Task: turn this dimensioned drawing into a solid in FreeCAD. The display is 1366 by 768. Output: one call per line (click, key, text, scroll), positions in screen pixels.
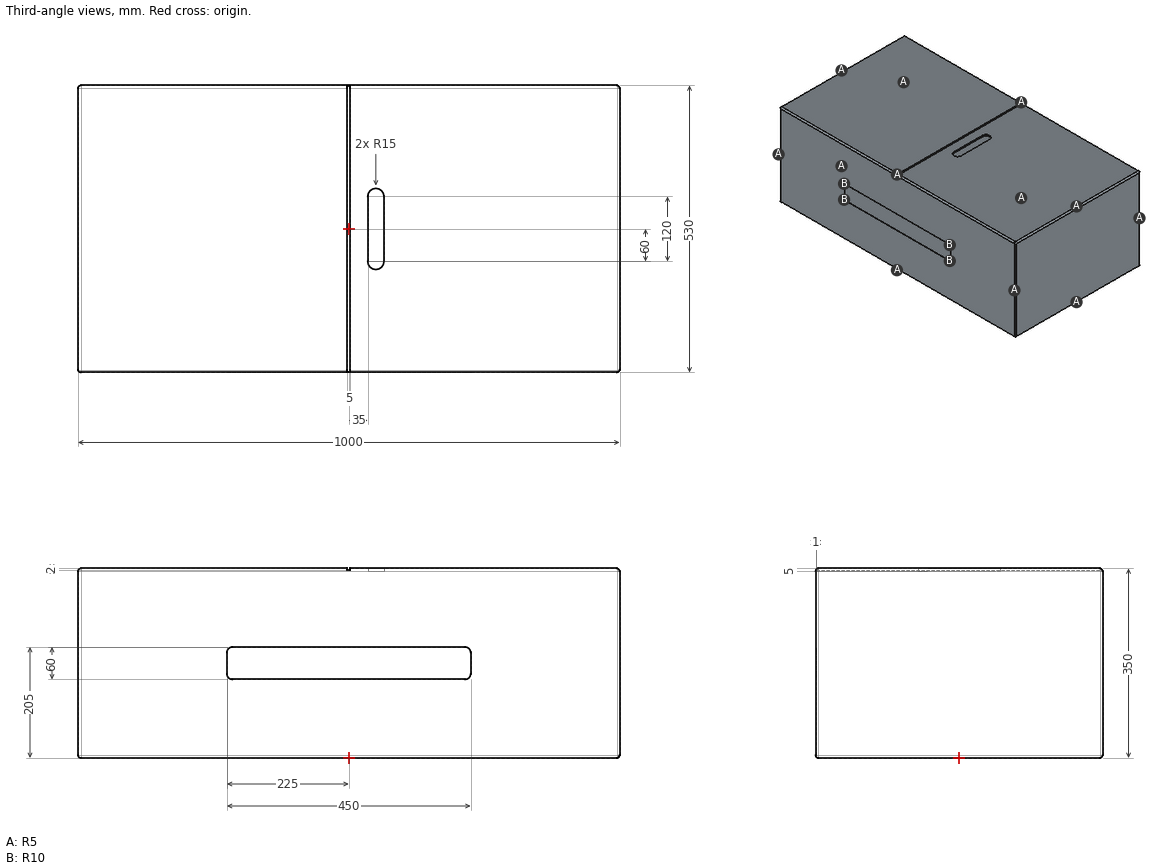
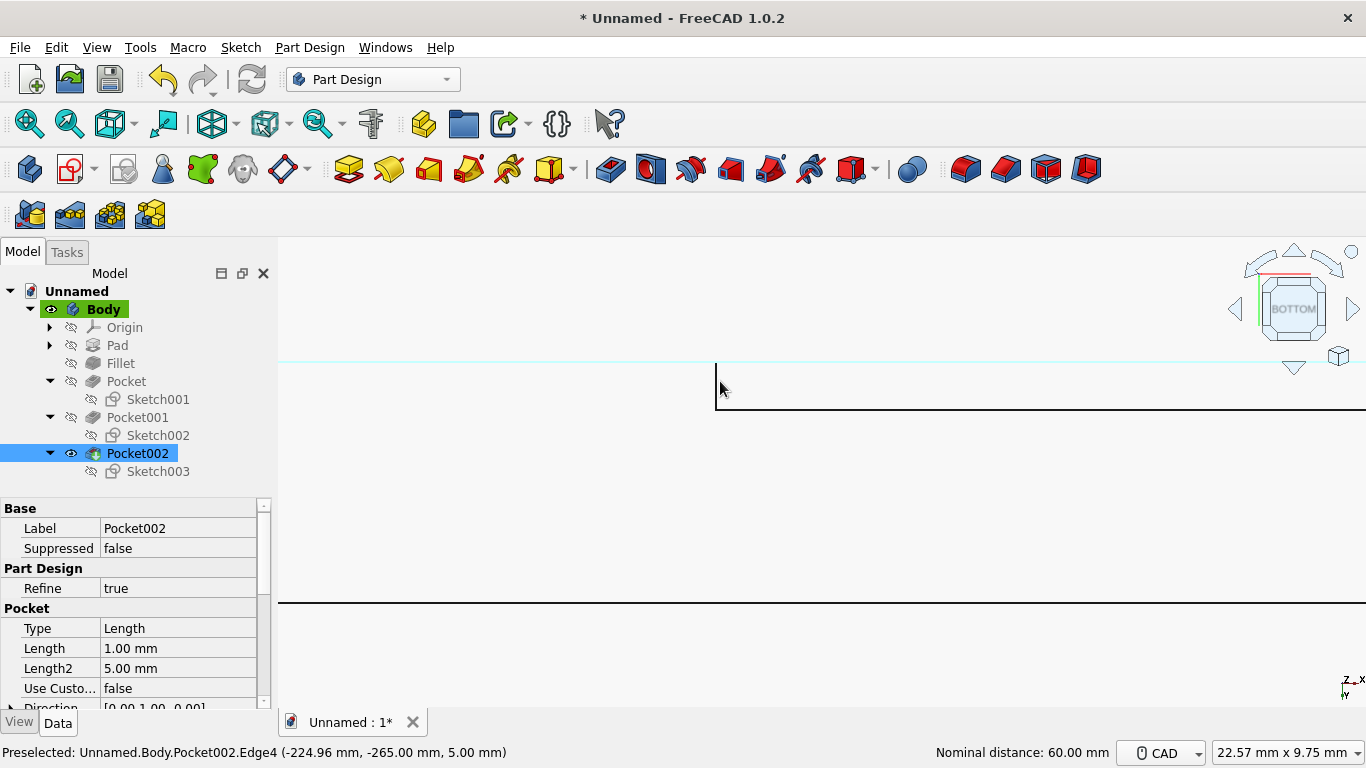
click(716, 385, ctrl)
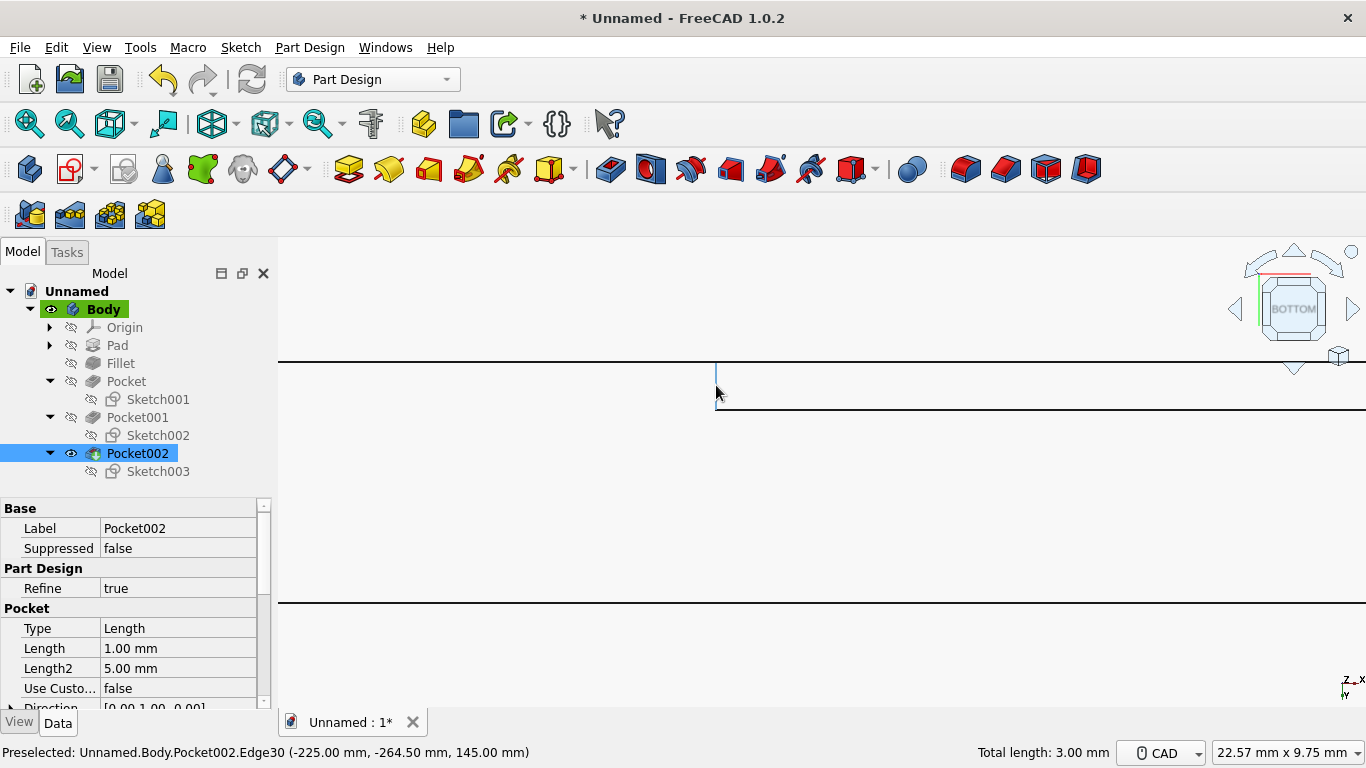
click(30, 124)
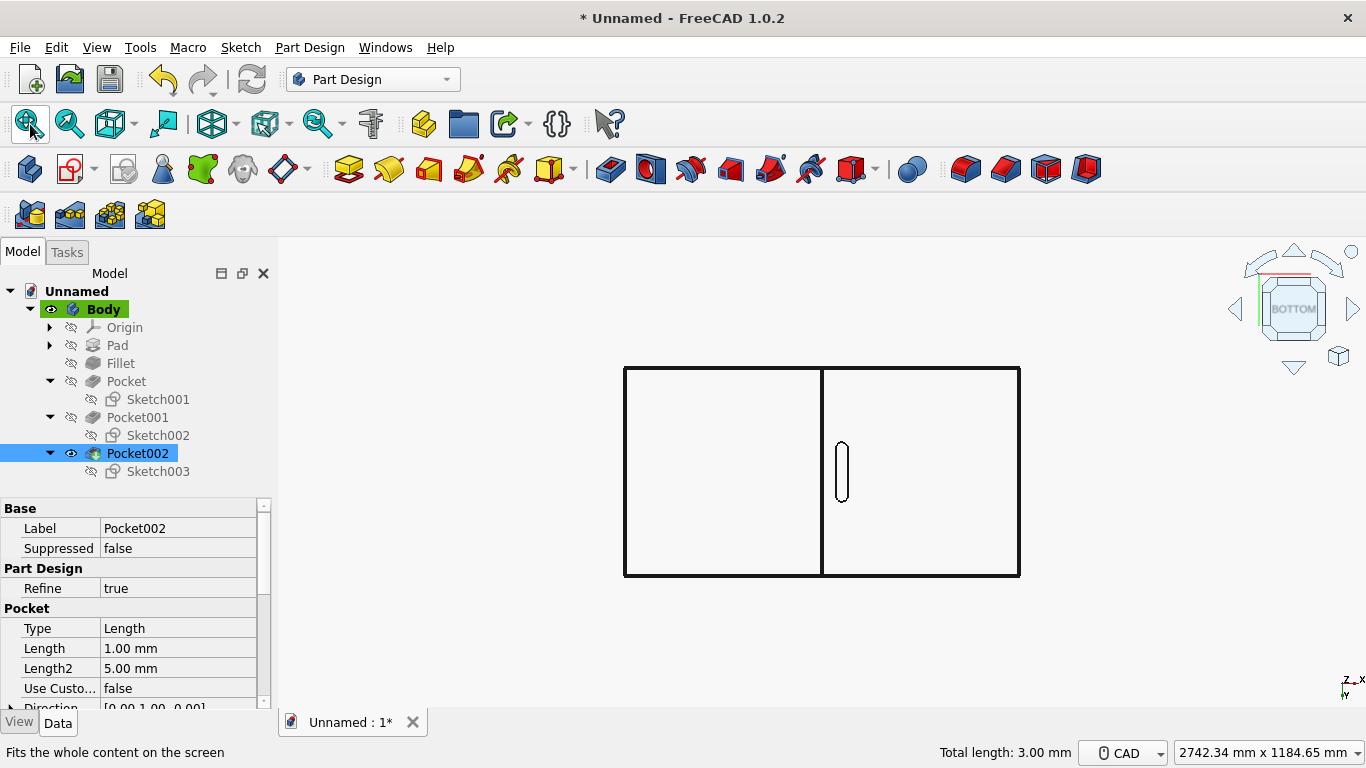
key(4)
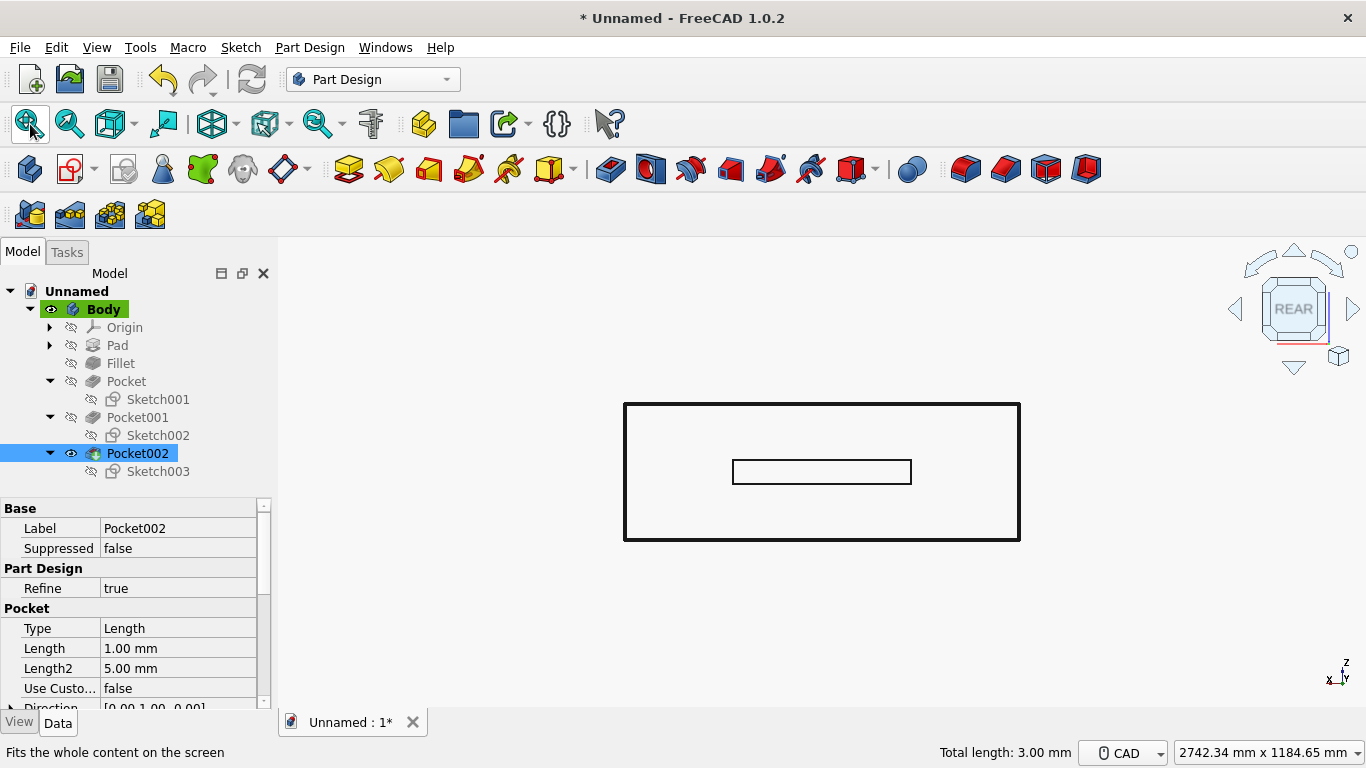
click(30, 124)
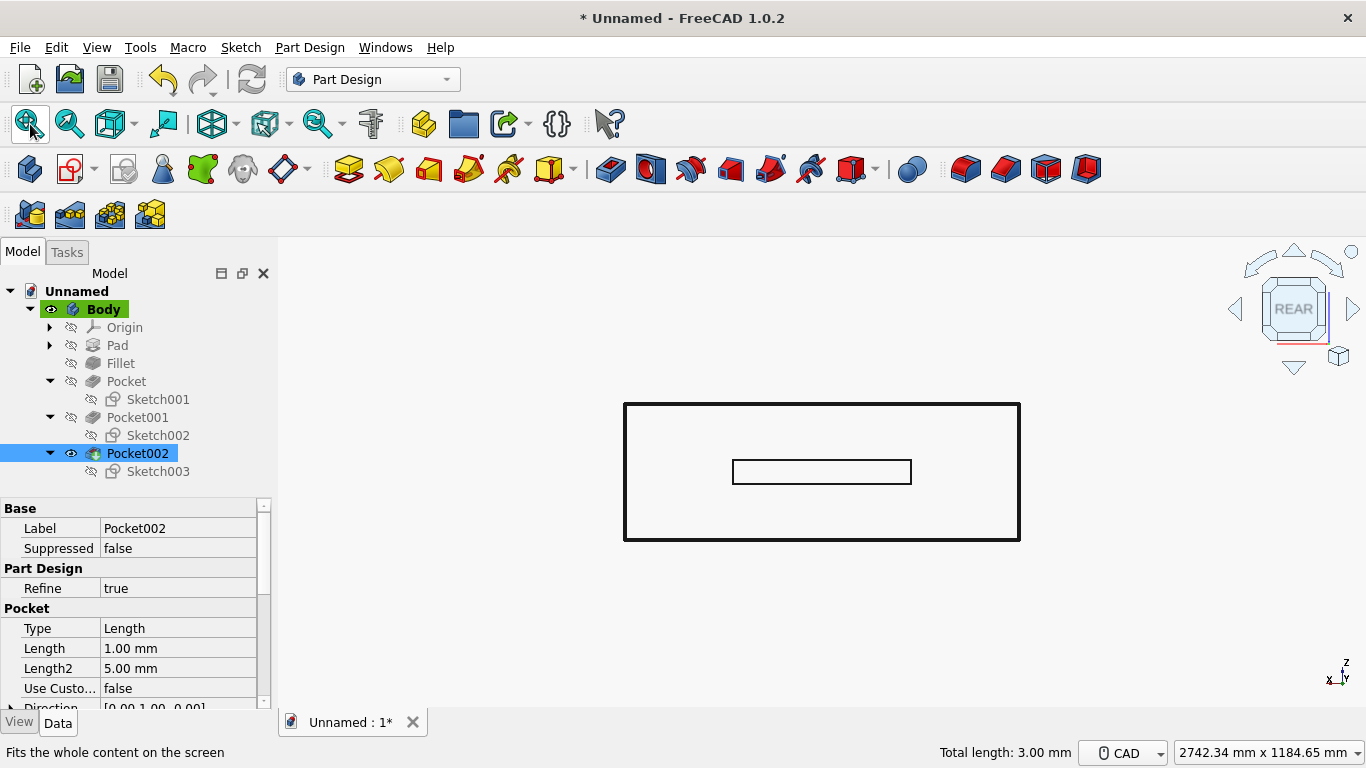
scroll(911, 459, up, 15)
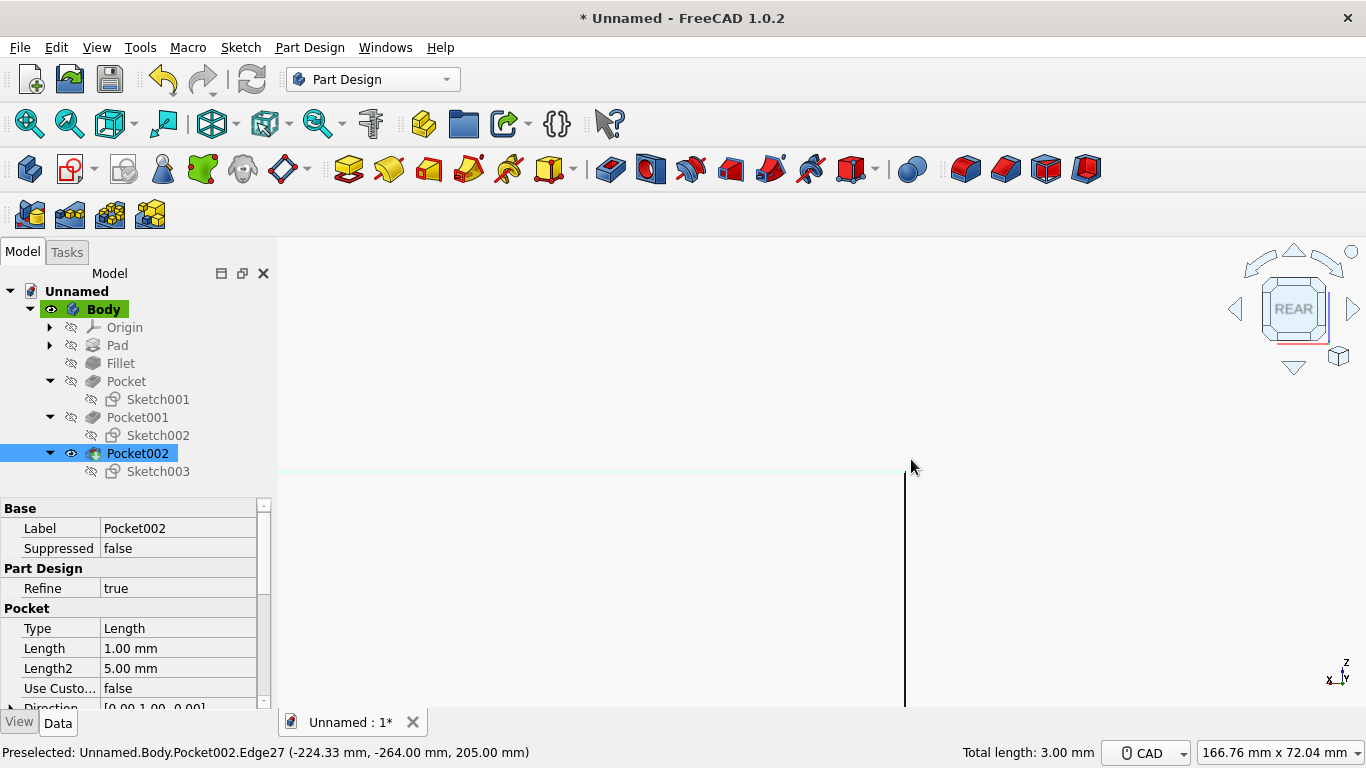
scroll(905, 471, up, 9)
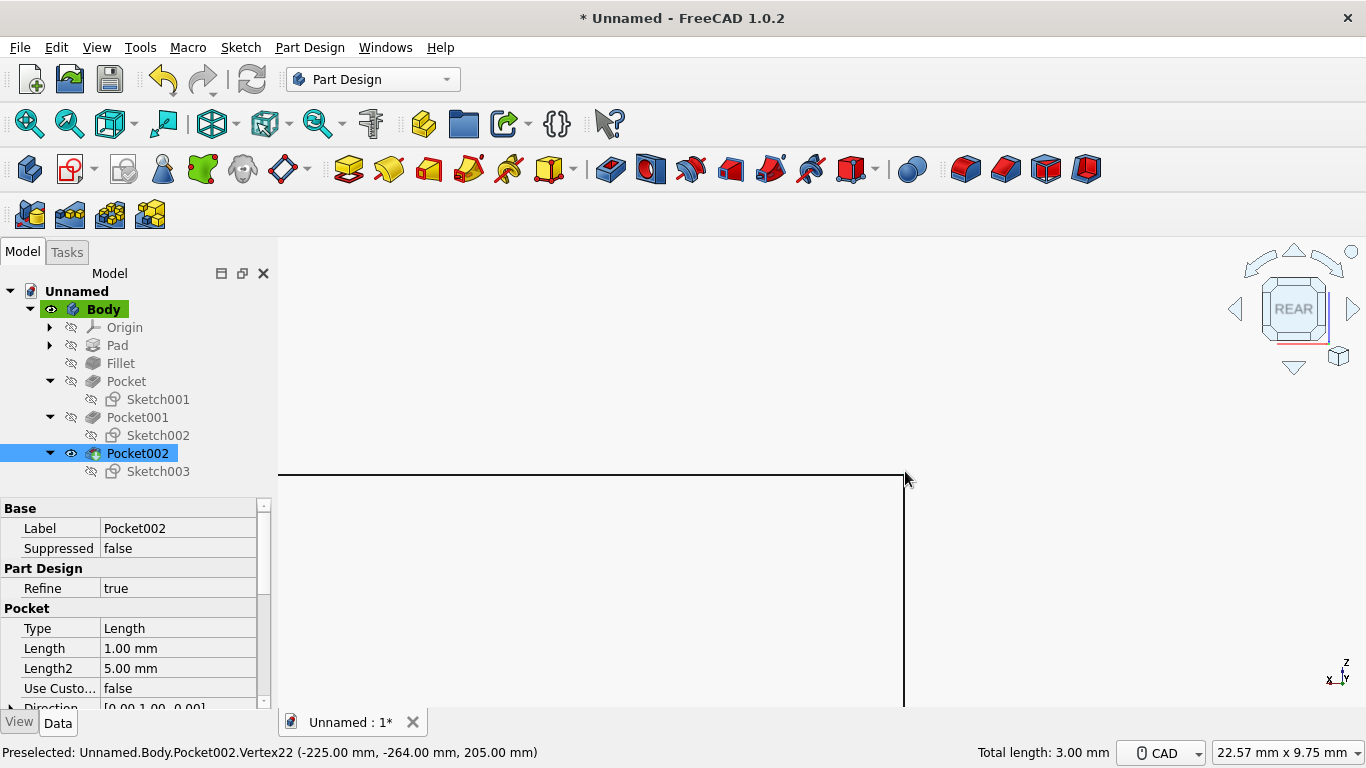
click(30, 124)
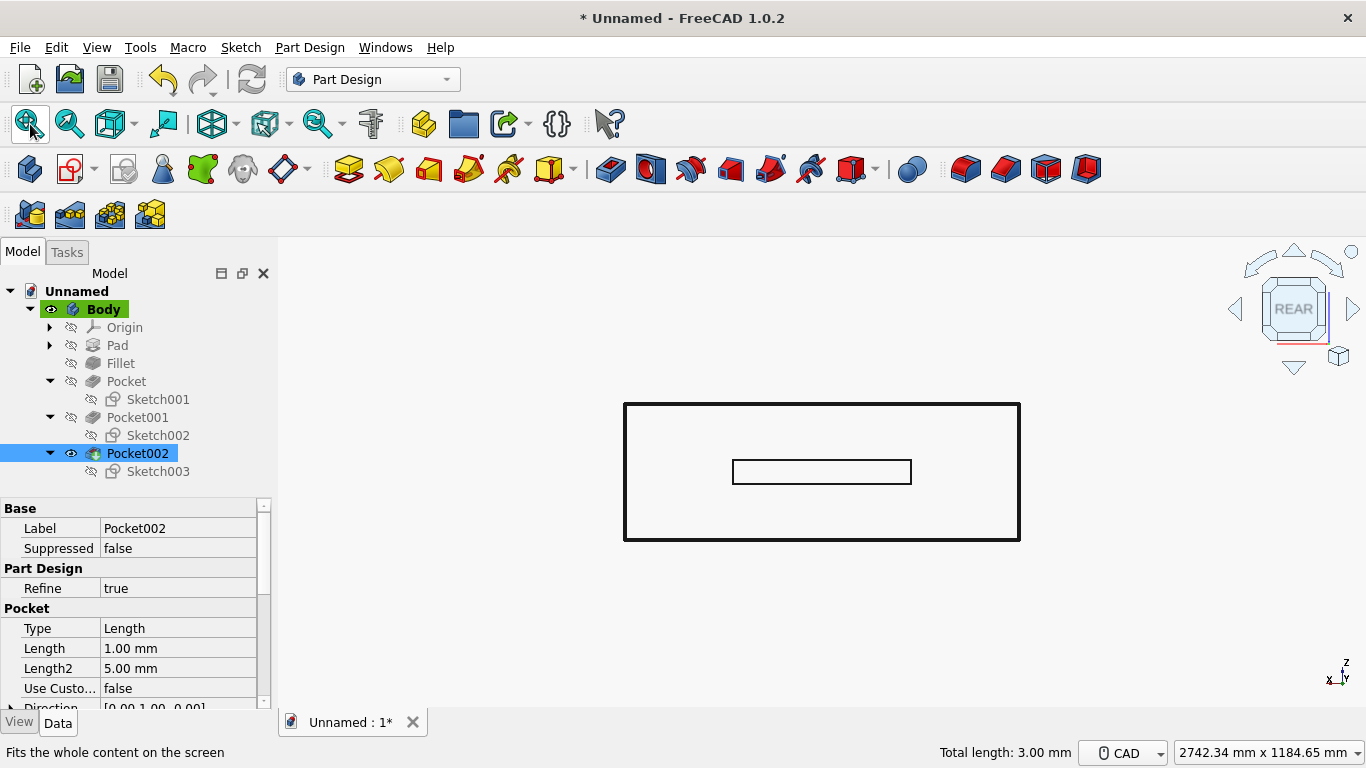
key(6)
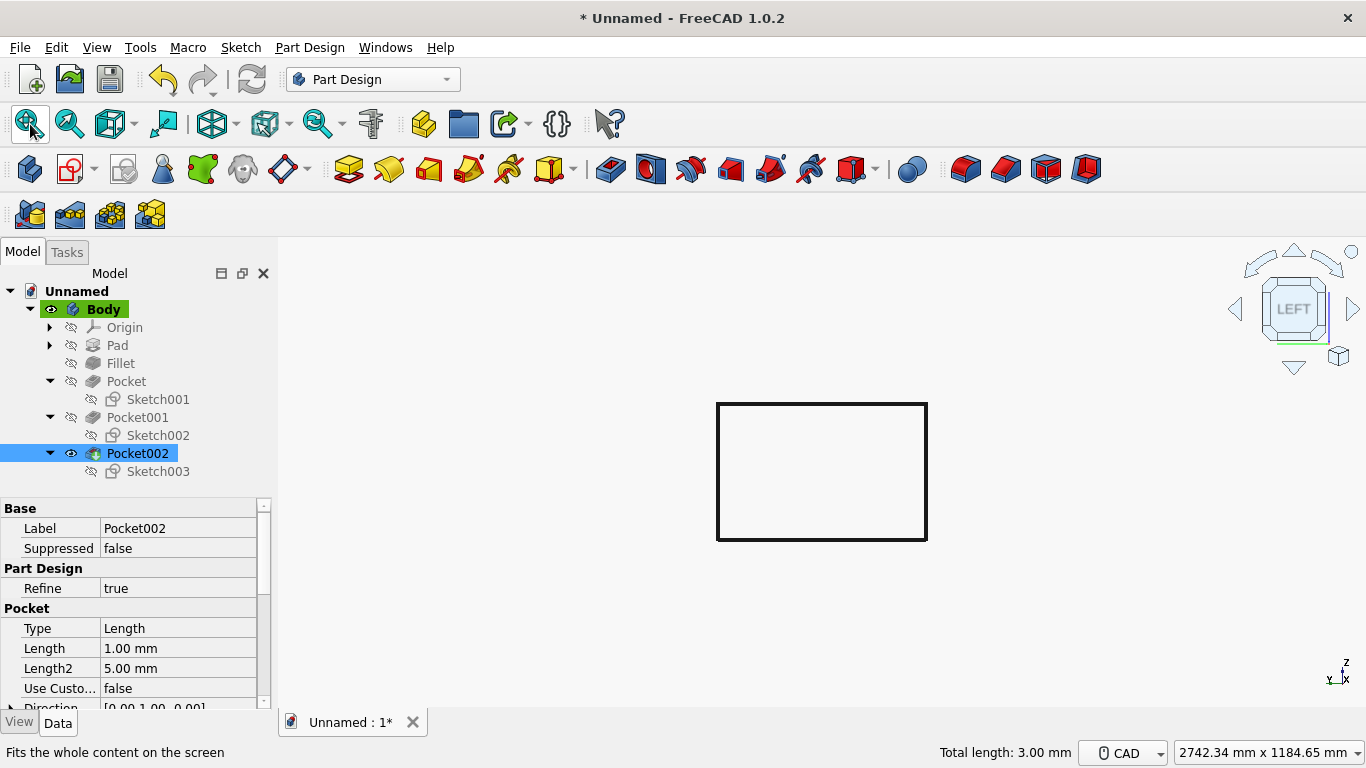
click(30, 124)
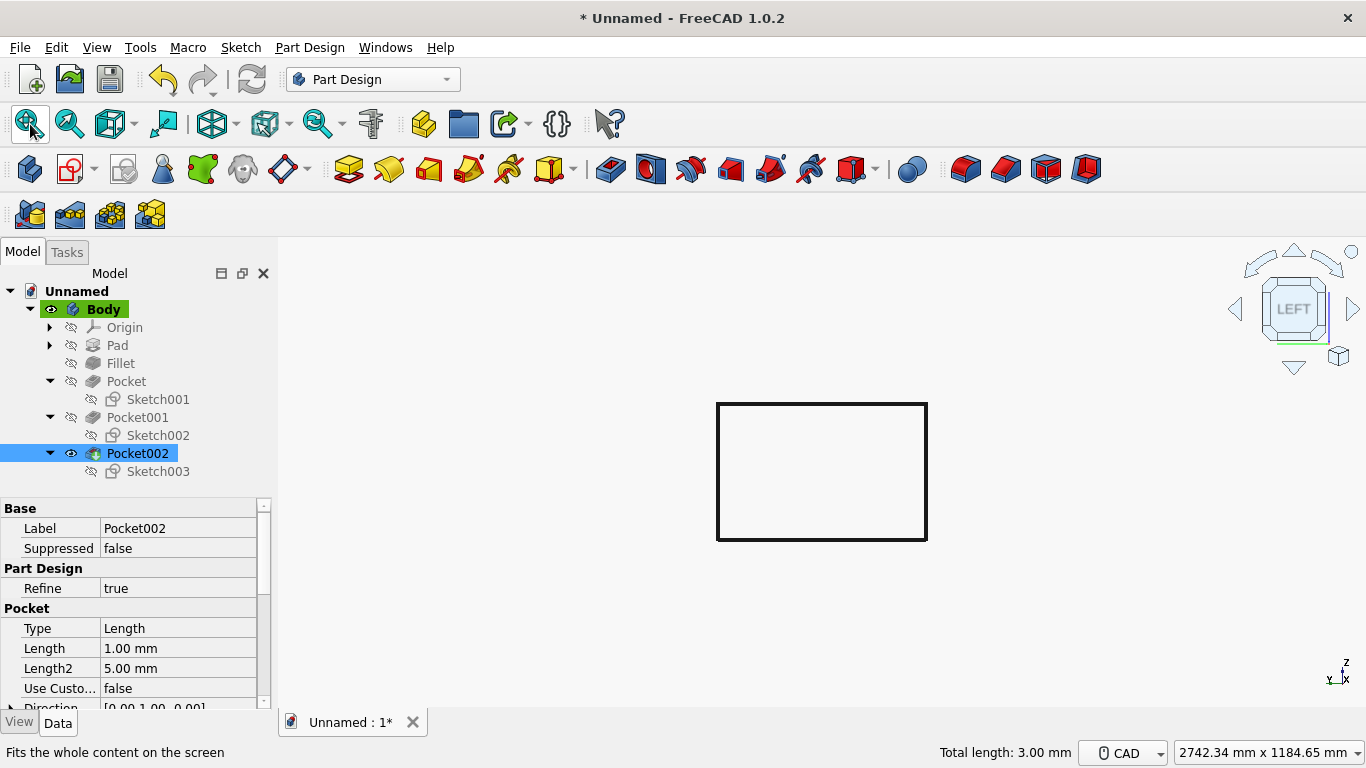
scroll(927, 459, up, 15)